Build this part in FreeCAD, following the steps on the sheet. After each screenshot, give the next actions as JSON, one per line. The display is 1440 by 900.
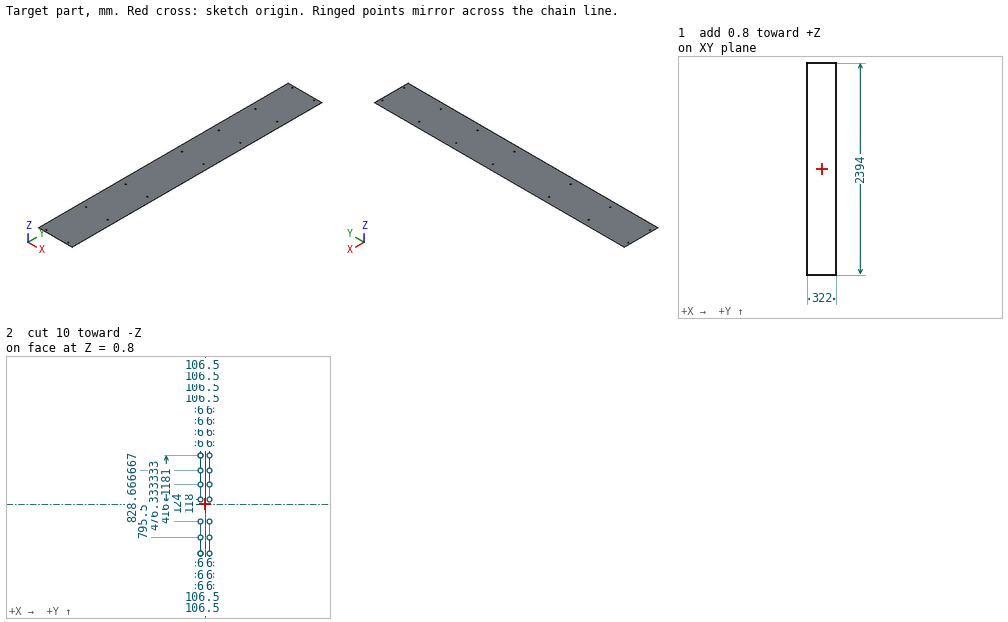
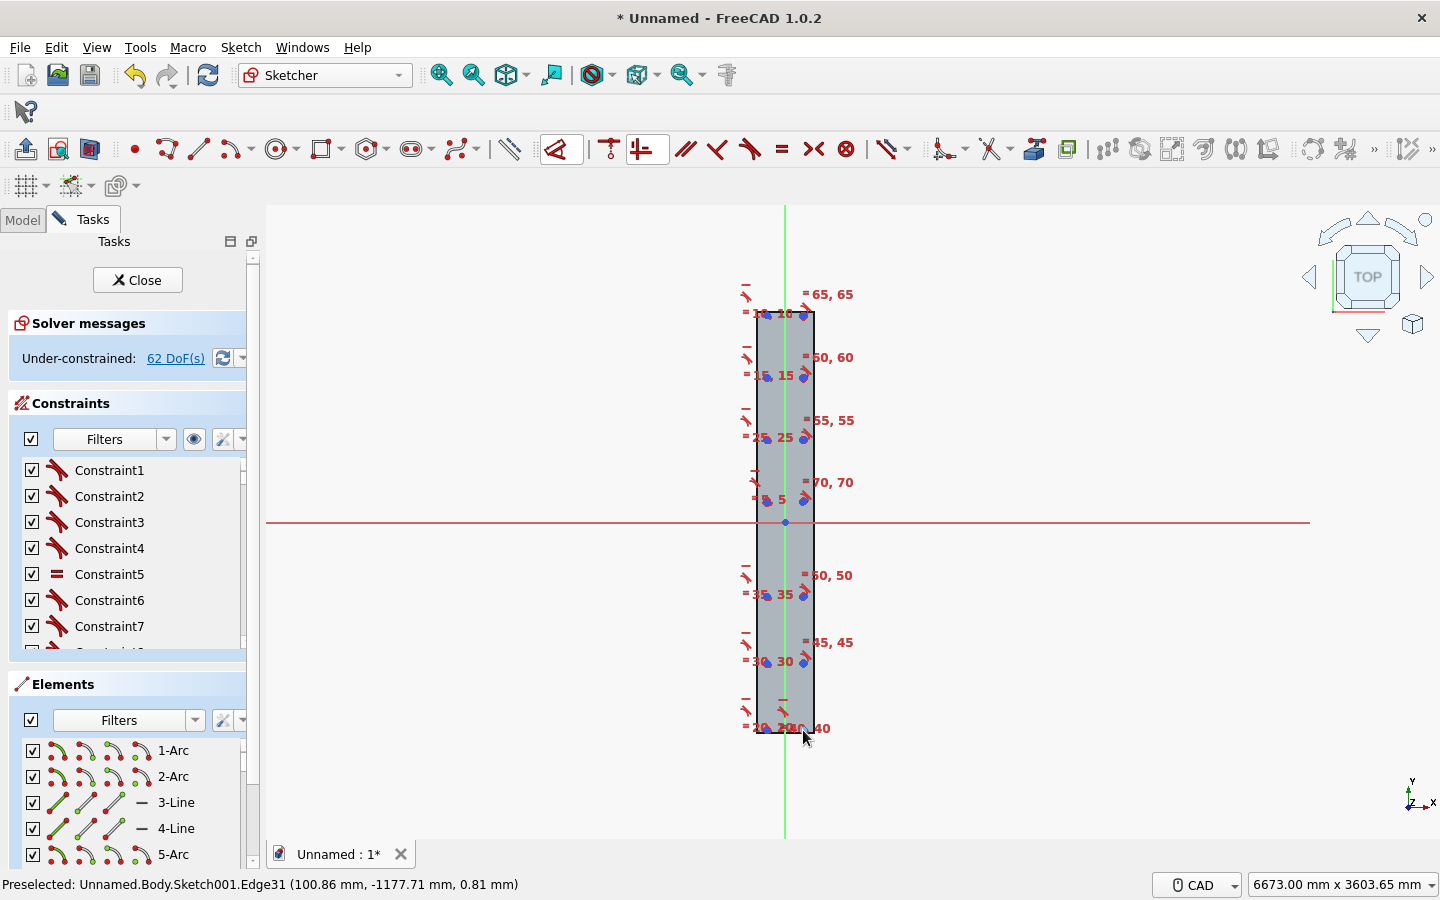
{"action": "scroll", "coordinate": [803, 663], "scroll_direction": "up", "scroll_amount": 14}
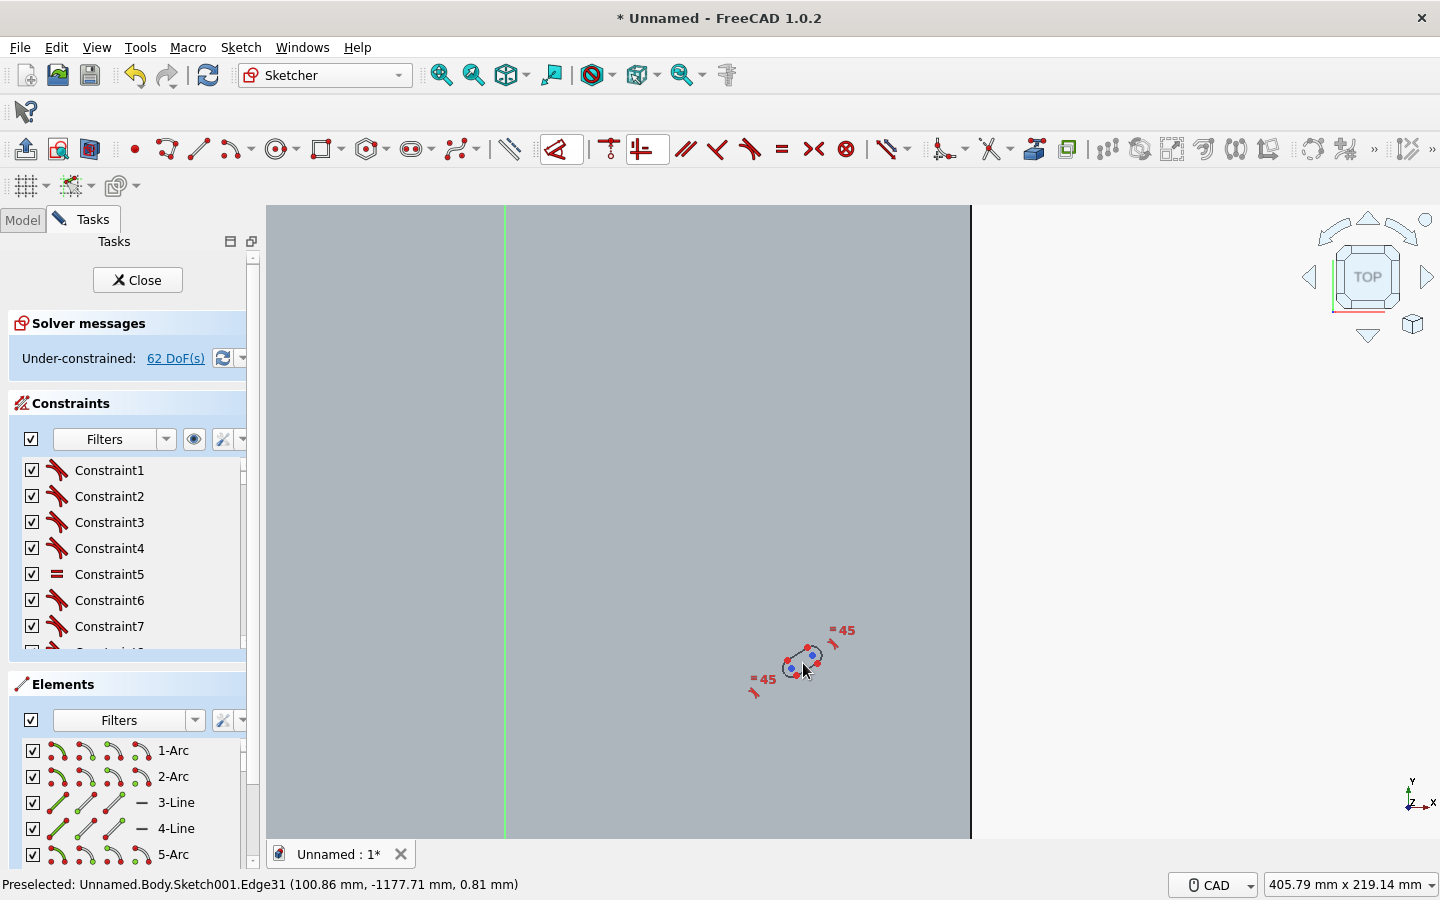
{"action": "left_click", "coordinate": [795, 655]}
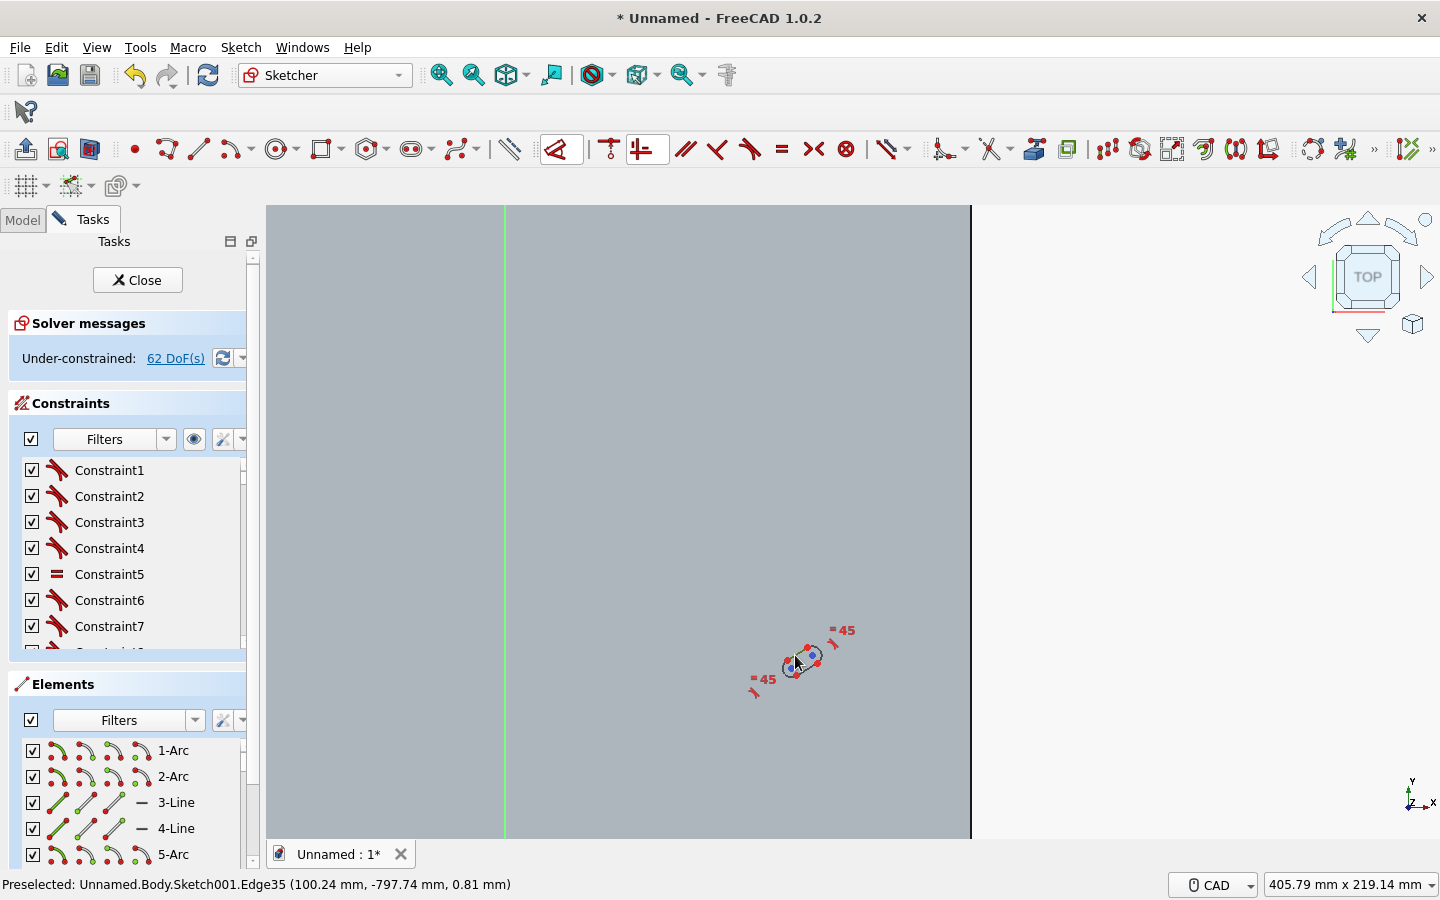
{"action": "key", "text": "h"}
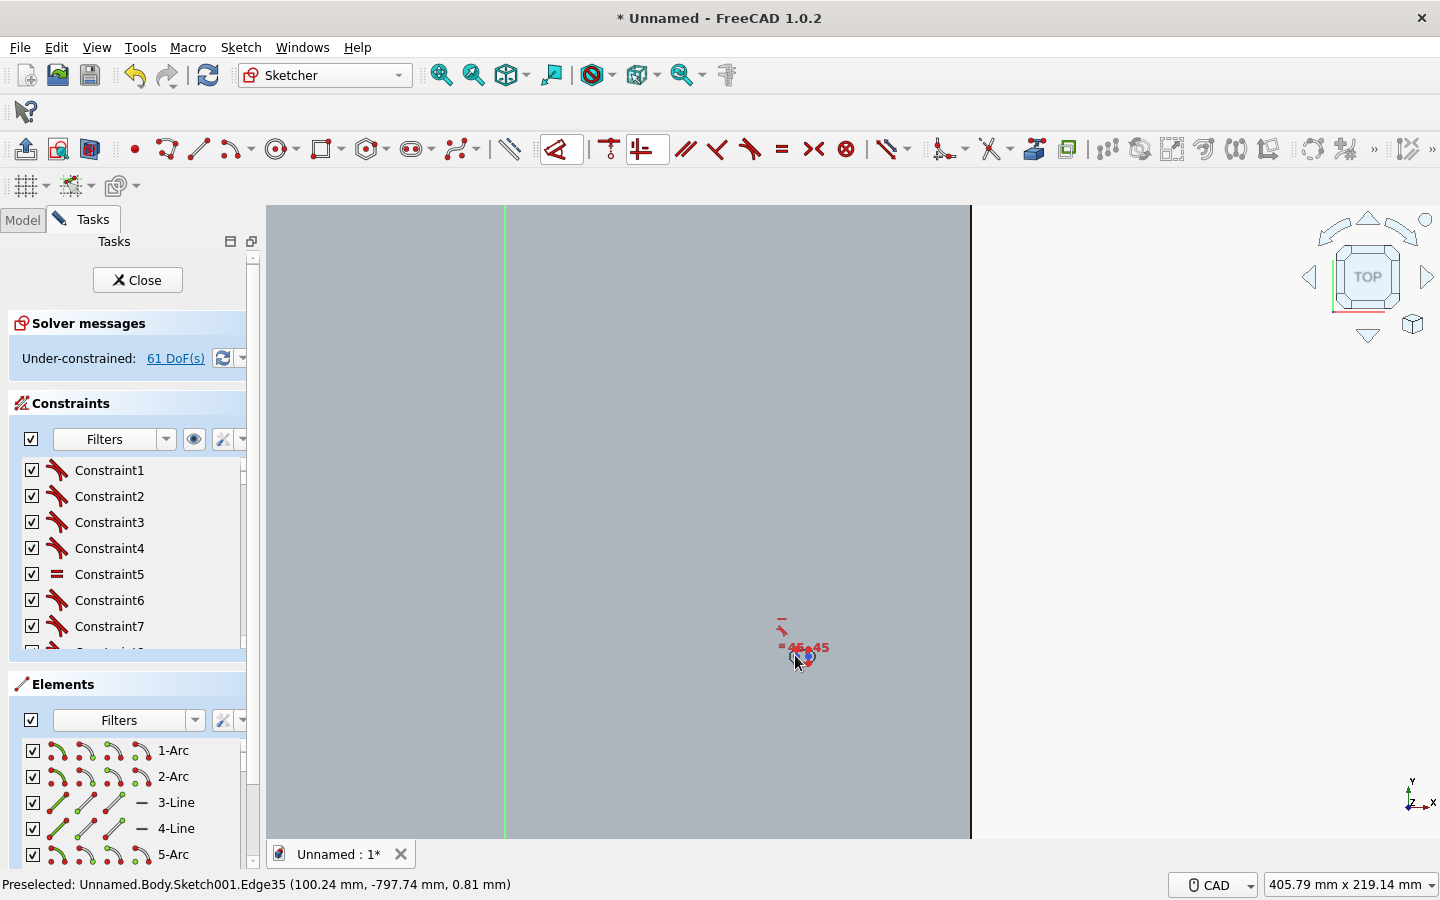
{"action": "scroll", "coordinate": [803, 663], "scroll_direction": "down", "scroll_amount": 14}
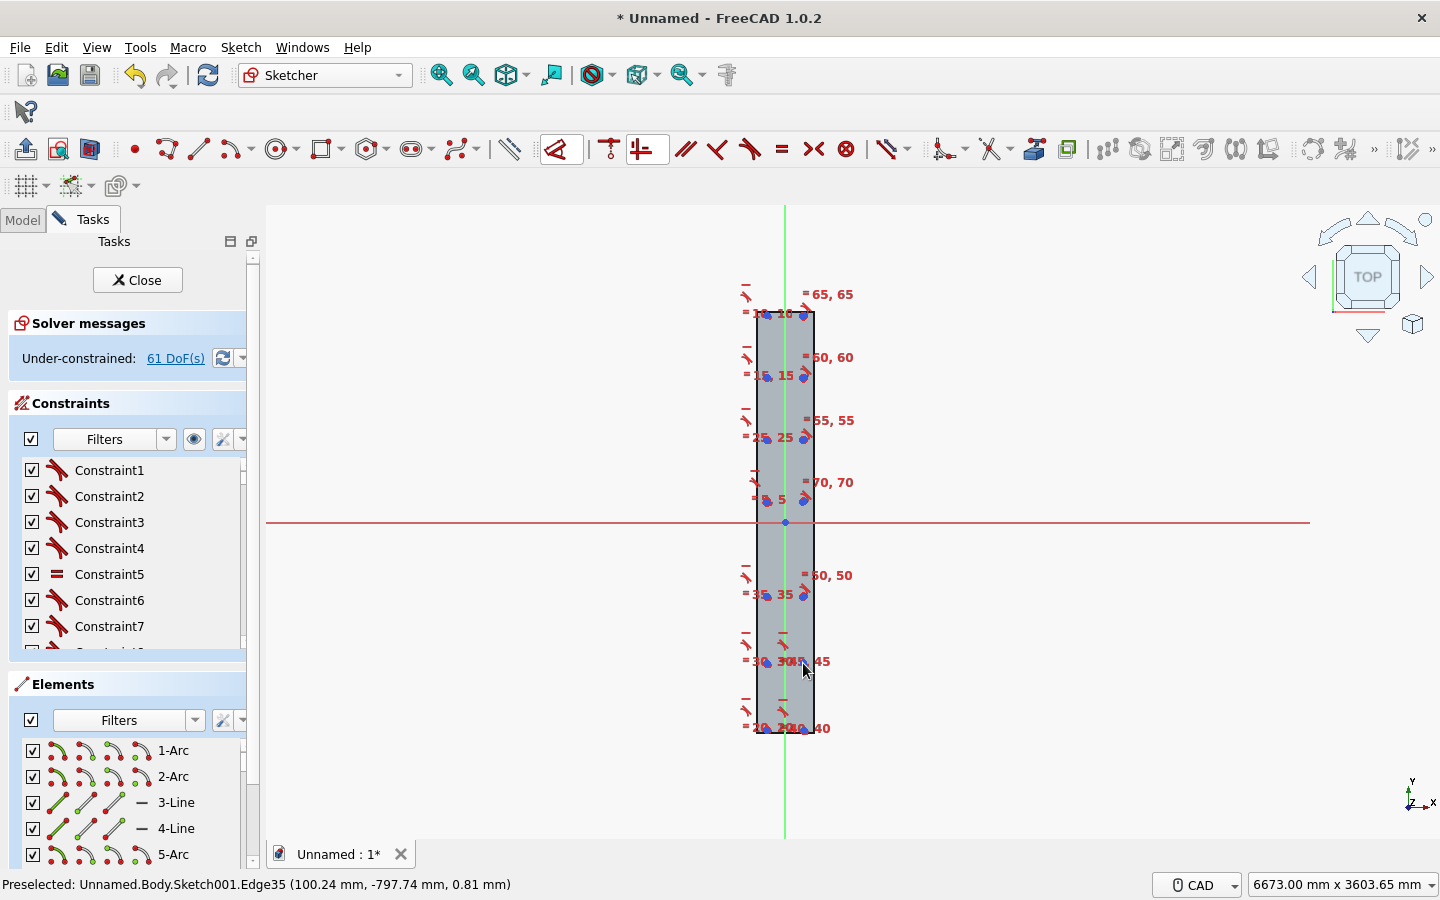
{"action": "scroll", "coordinate": [803, 596], "scroll_direction": "up", "scroll_amount": 14}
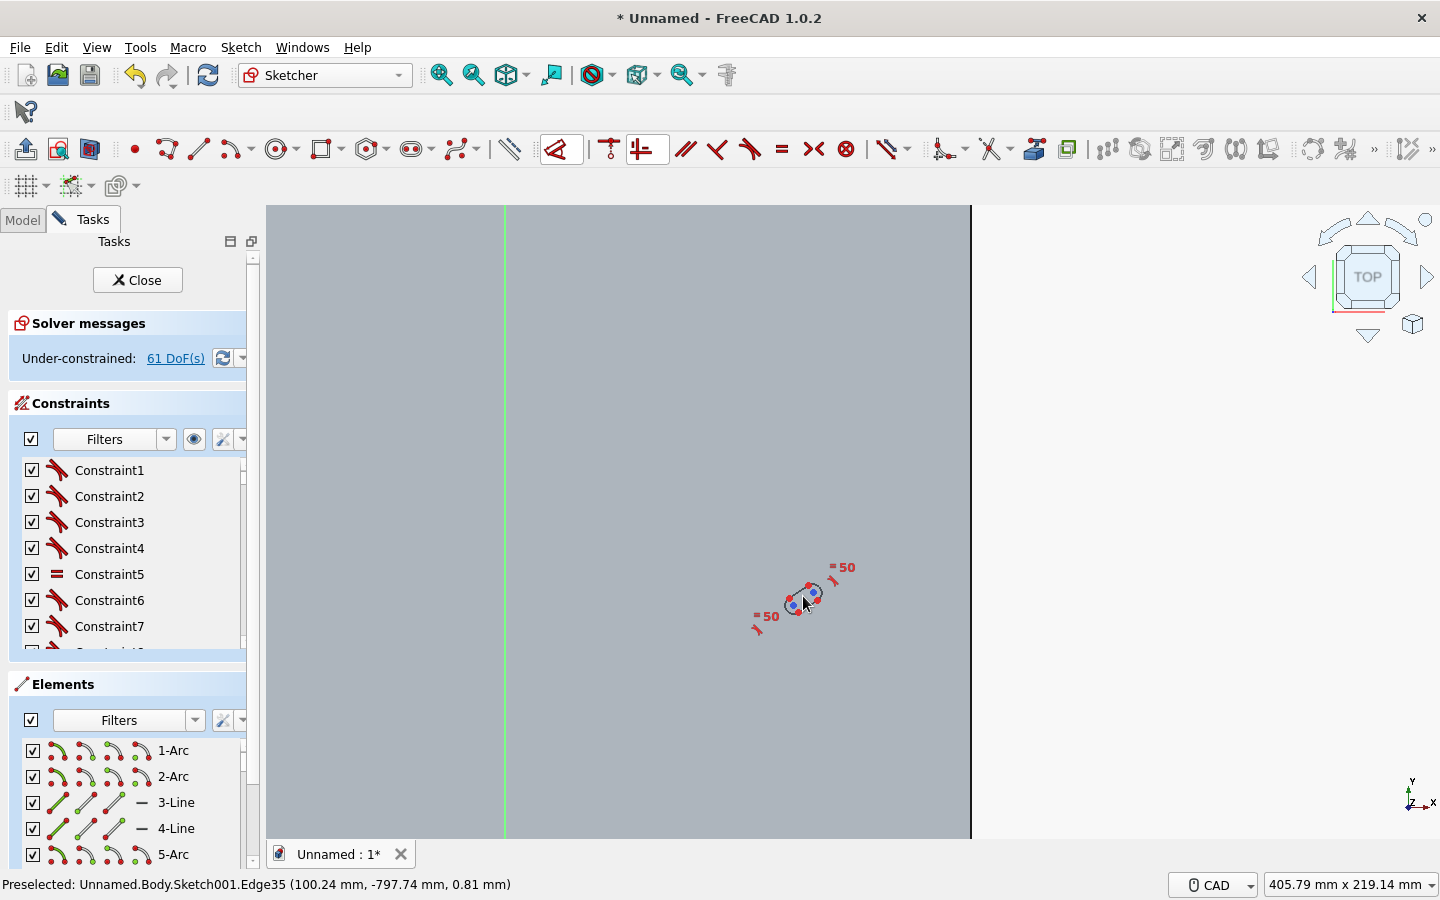
{"action": "left_click", "coordinate": [797, 593]}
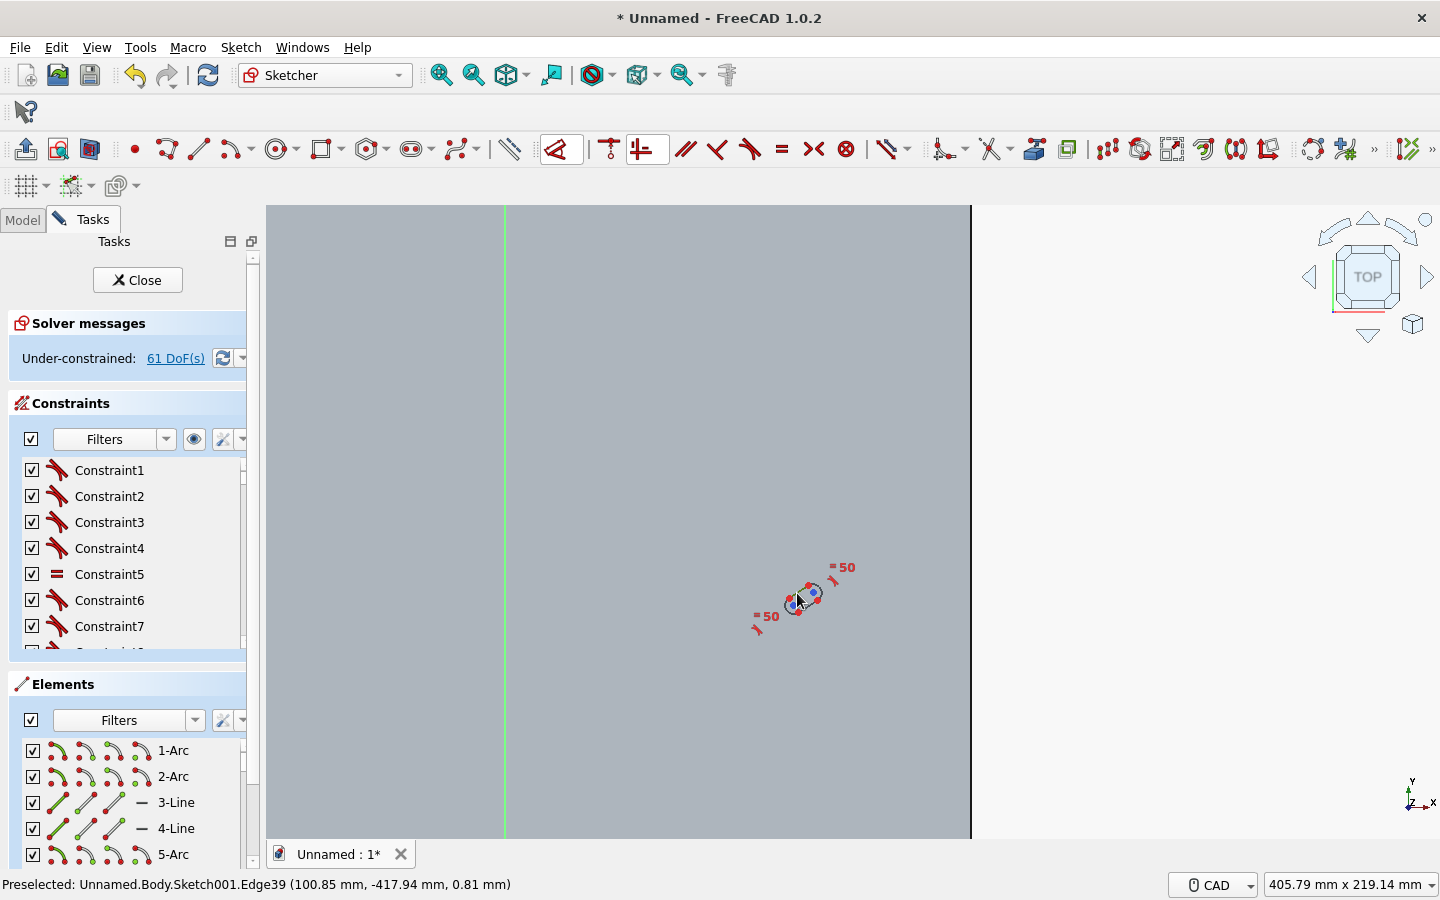
{"action": "key", "text": "h"}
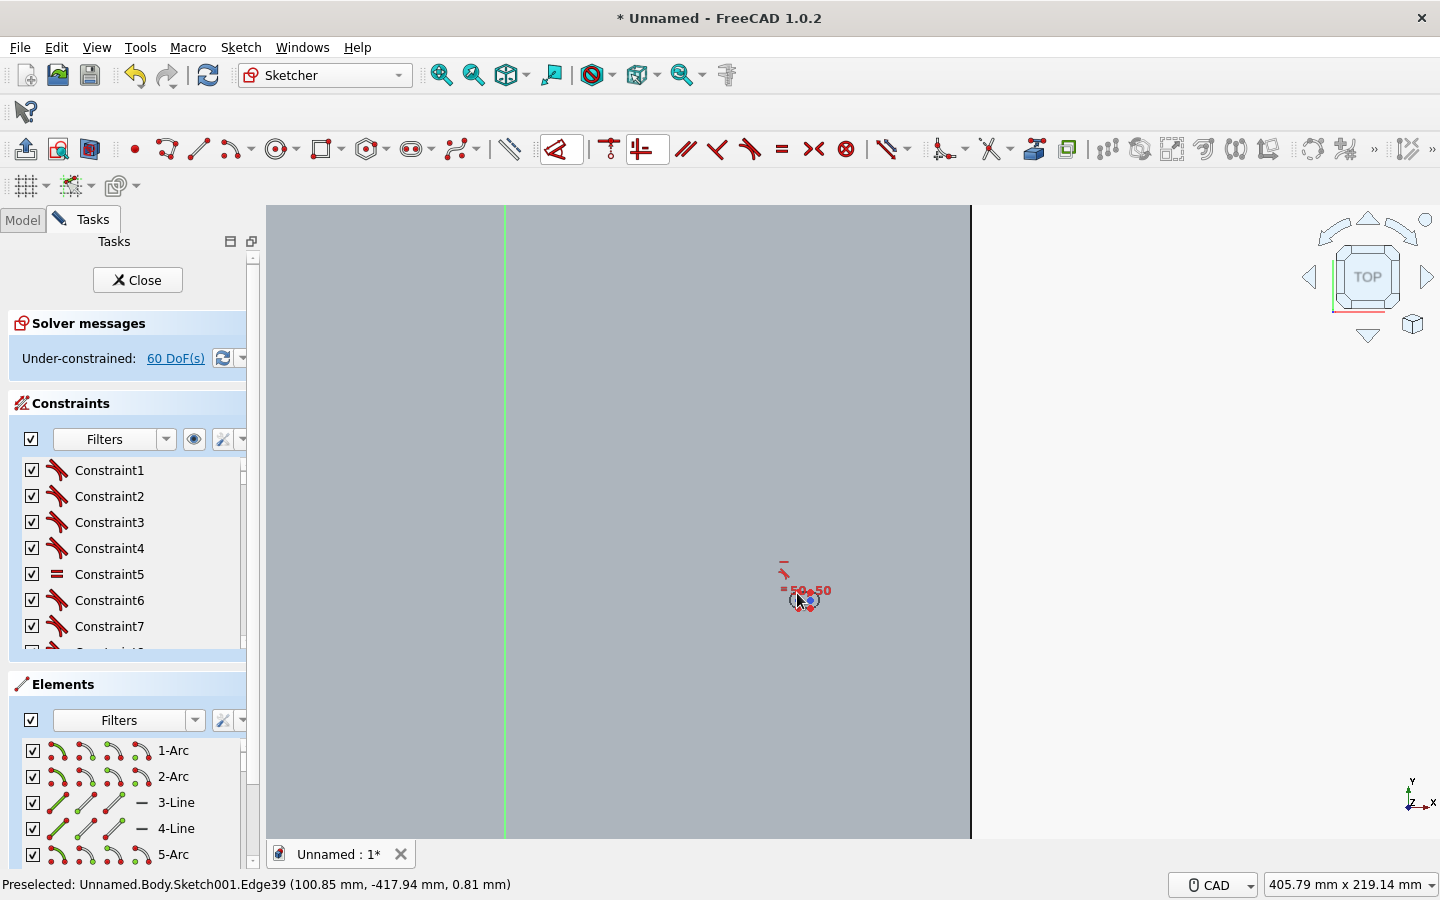
{"action": "scroll", "coordinate": [803, 596], "scroll_direction": "down", "scroll_amount": 14}